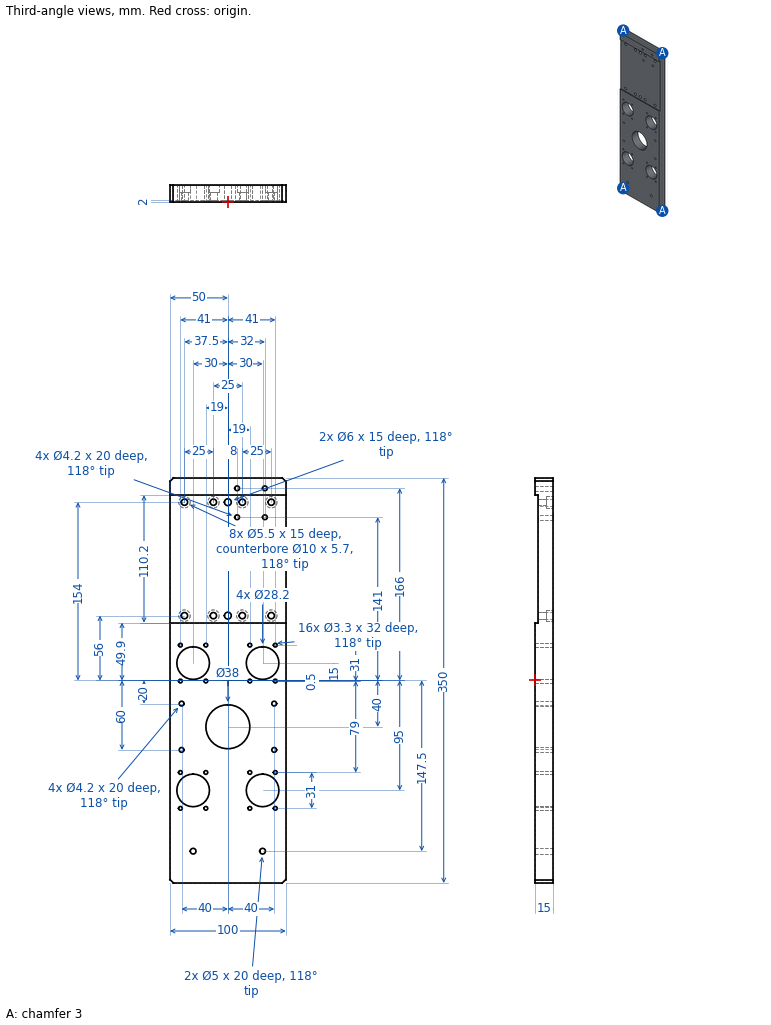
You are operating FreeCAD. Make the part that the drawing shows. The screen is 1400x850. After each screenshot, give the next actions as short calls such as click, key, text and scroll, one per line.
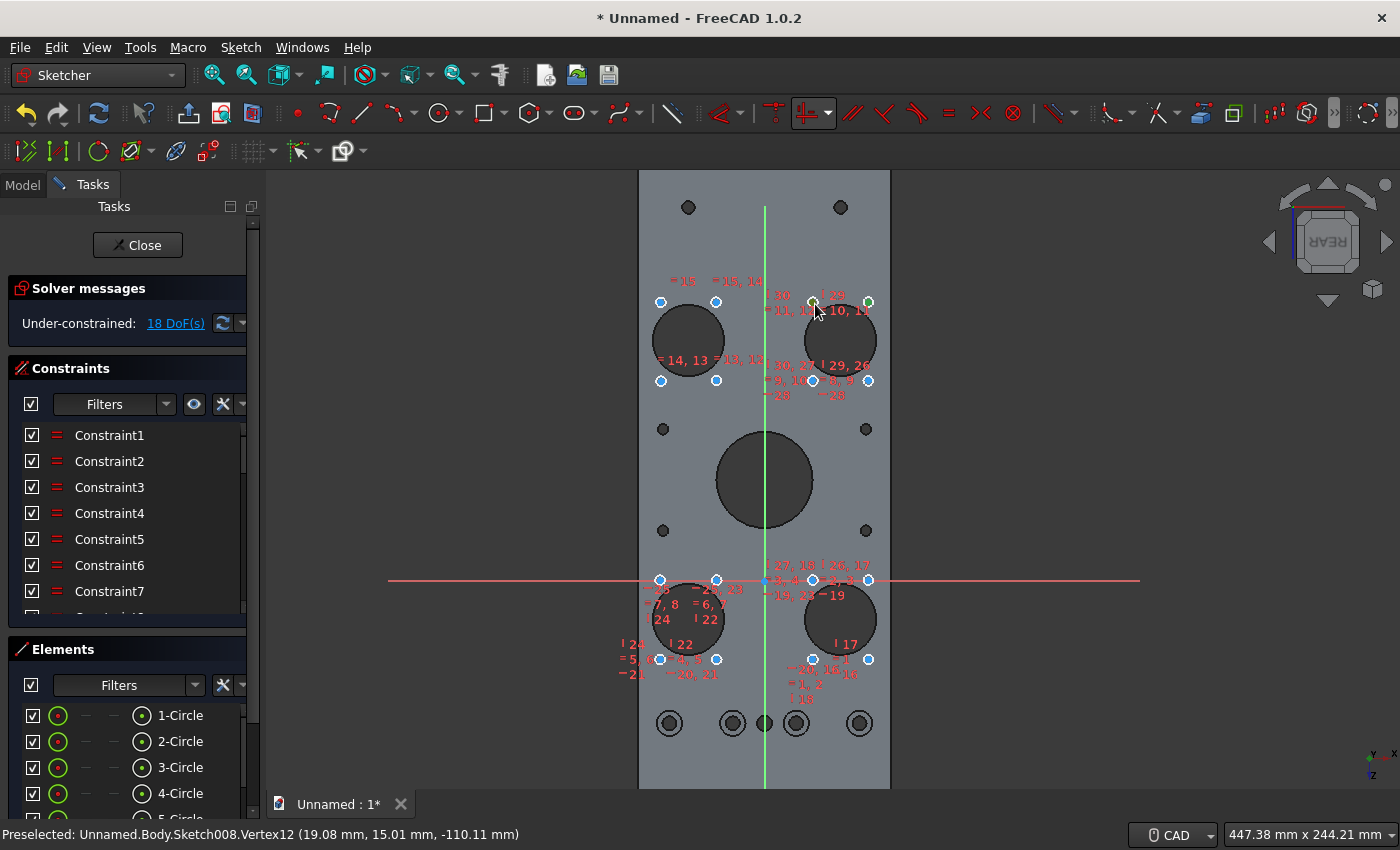
key(h)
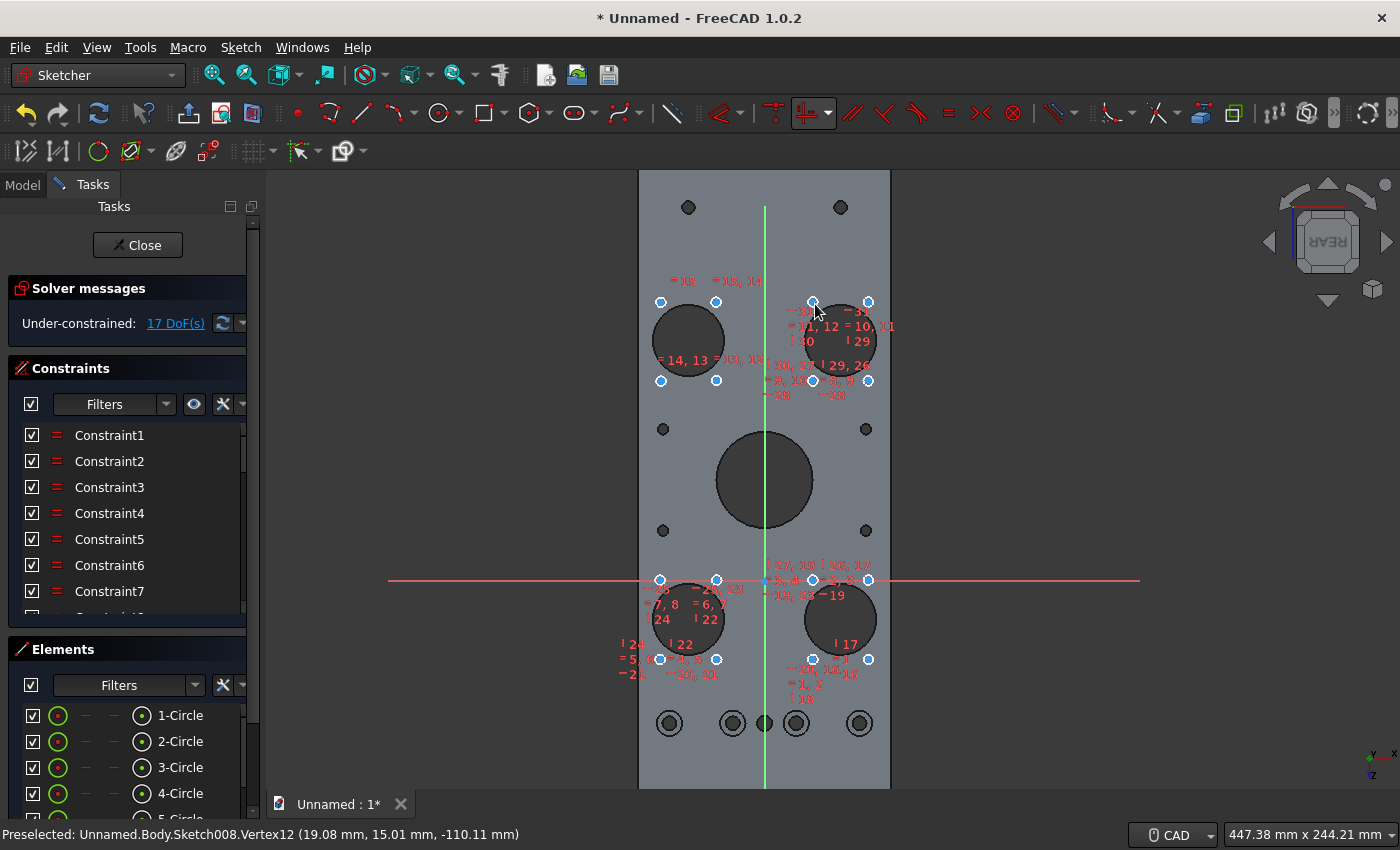
click(717, 580)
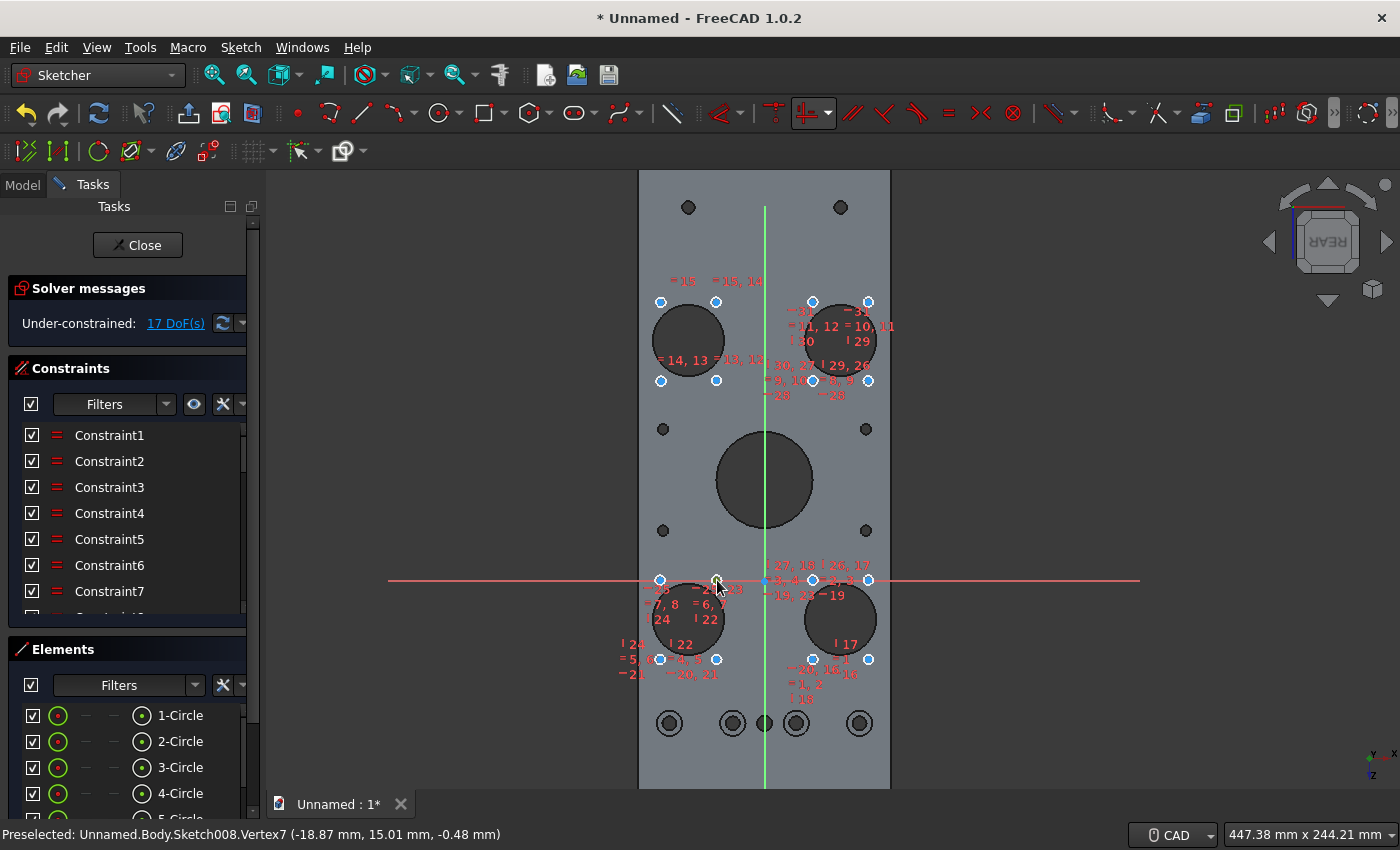
click(717, 380)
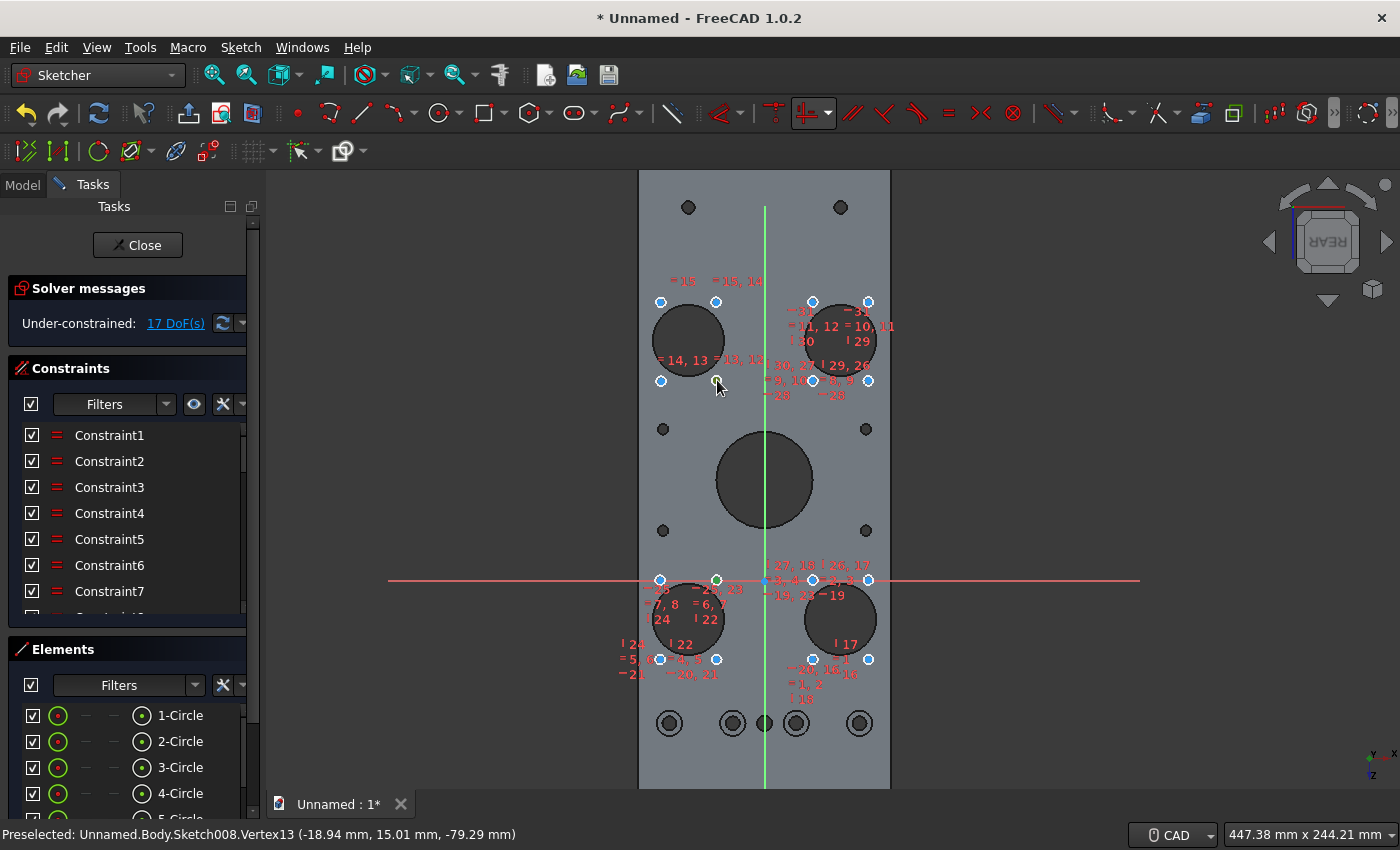
key(v)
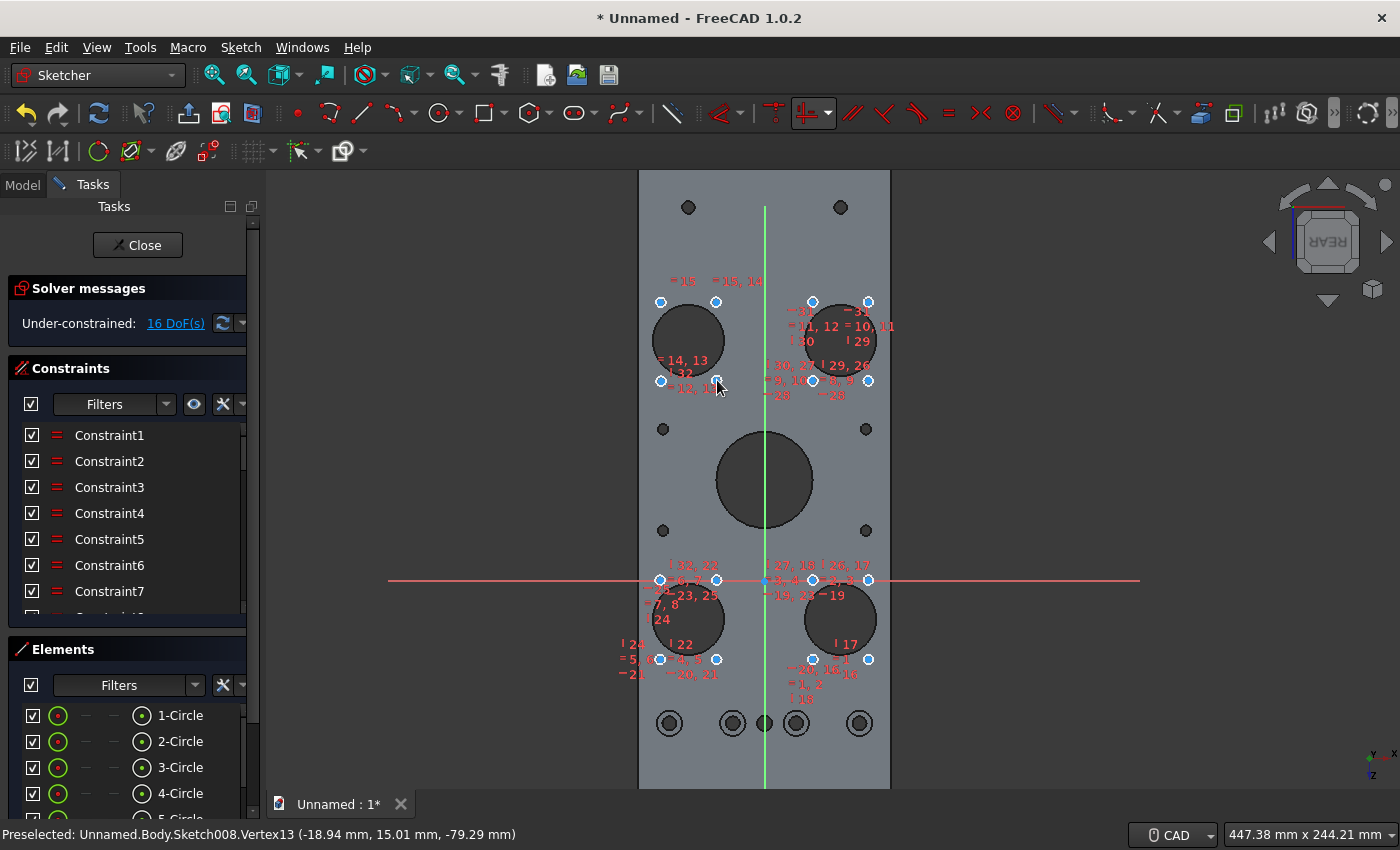
click(813, 381)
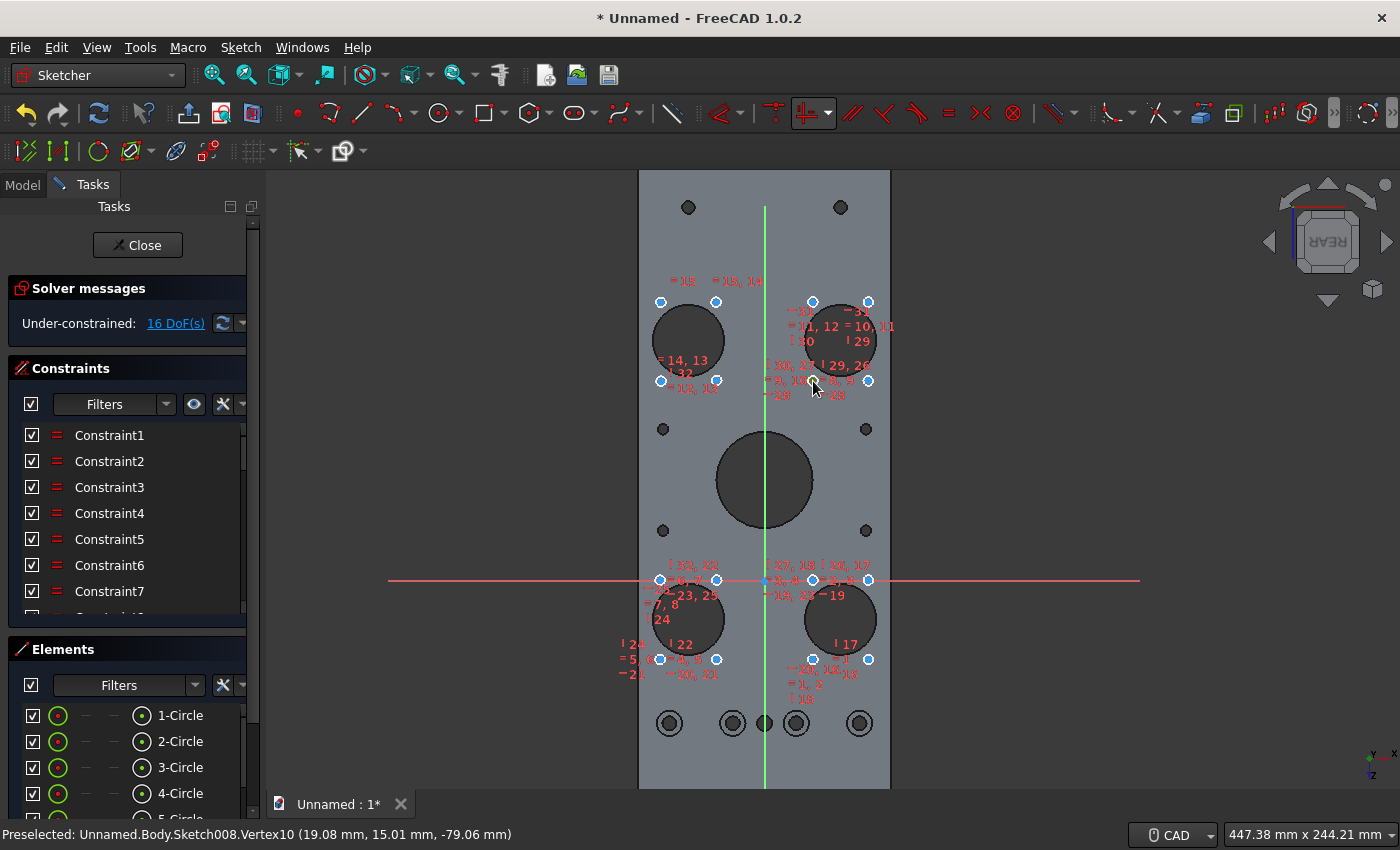
click(719, 382)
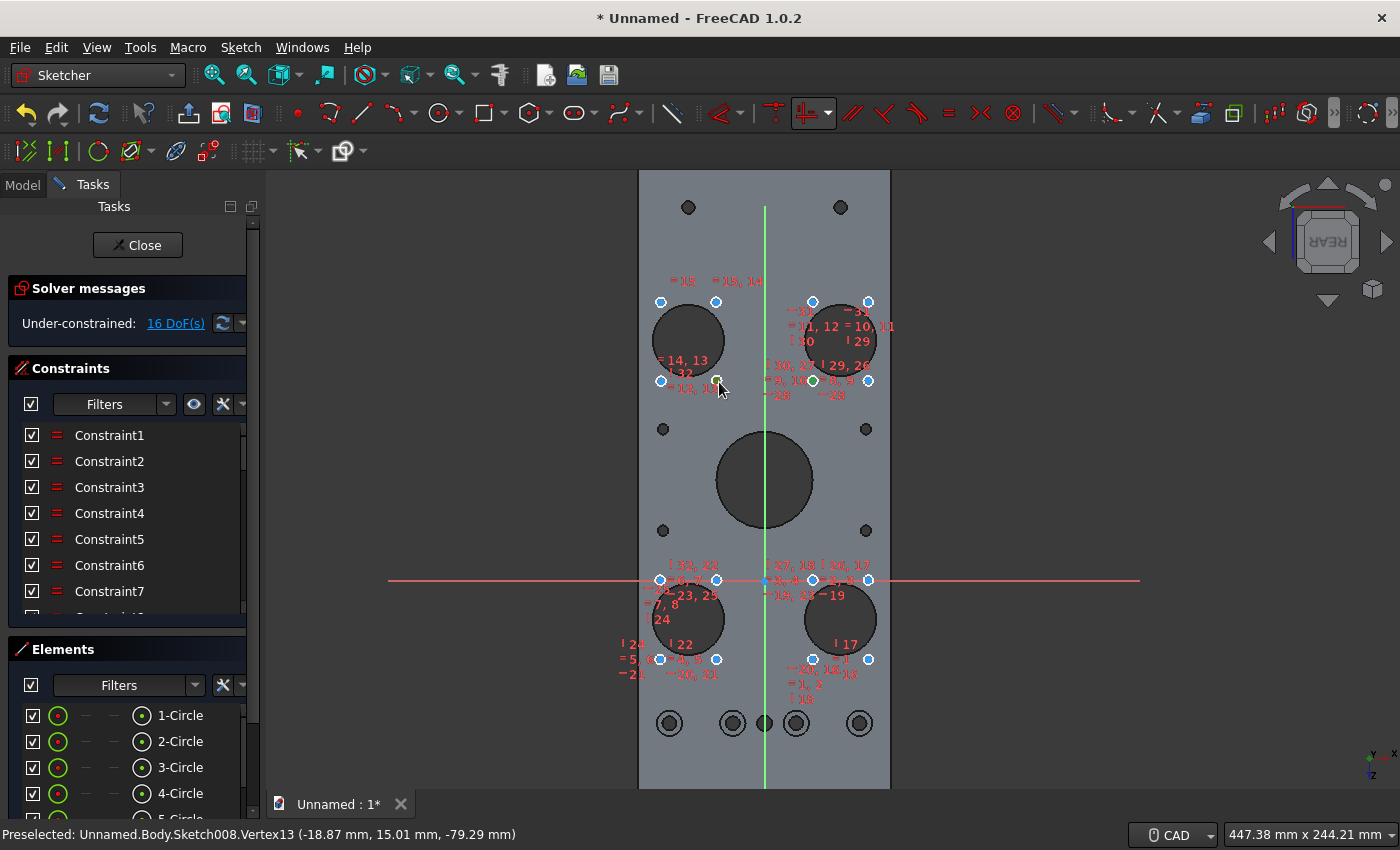
key(h)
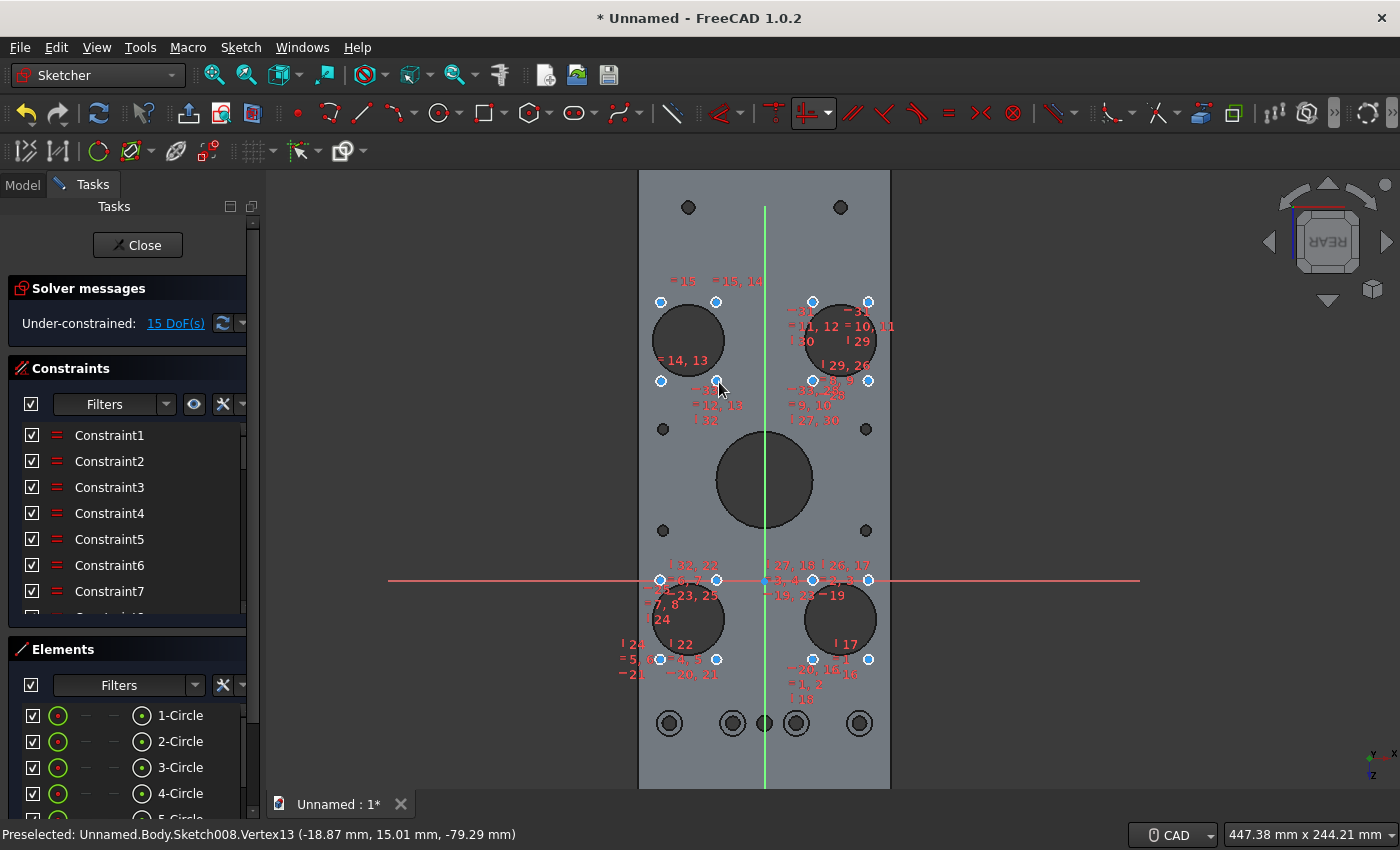
click(660, 580)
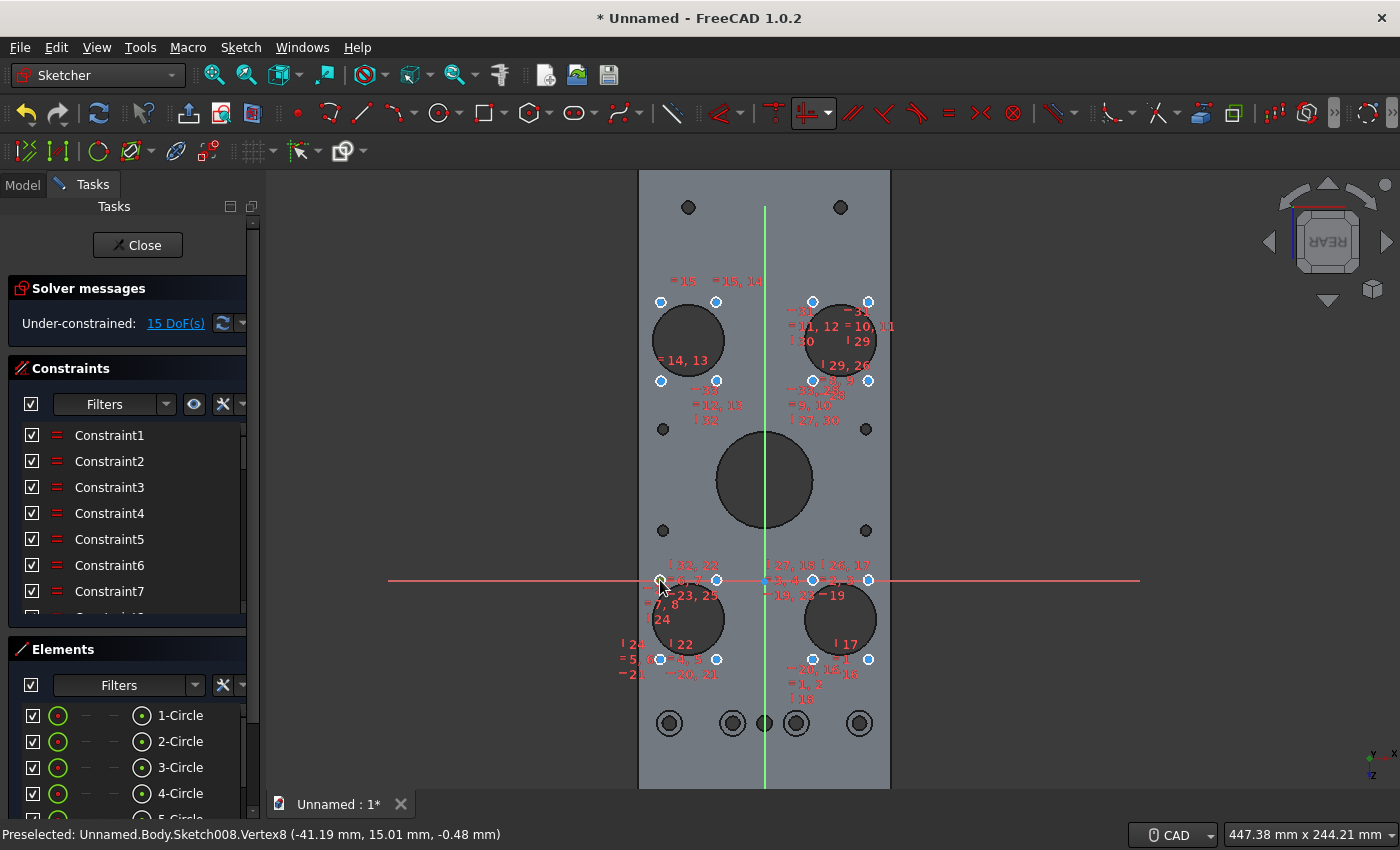
click(661, 381)